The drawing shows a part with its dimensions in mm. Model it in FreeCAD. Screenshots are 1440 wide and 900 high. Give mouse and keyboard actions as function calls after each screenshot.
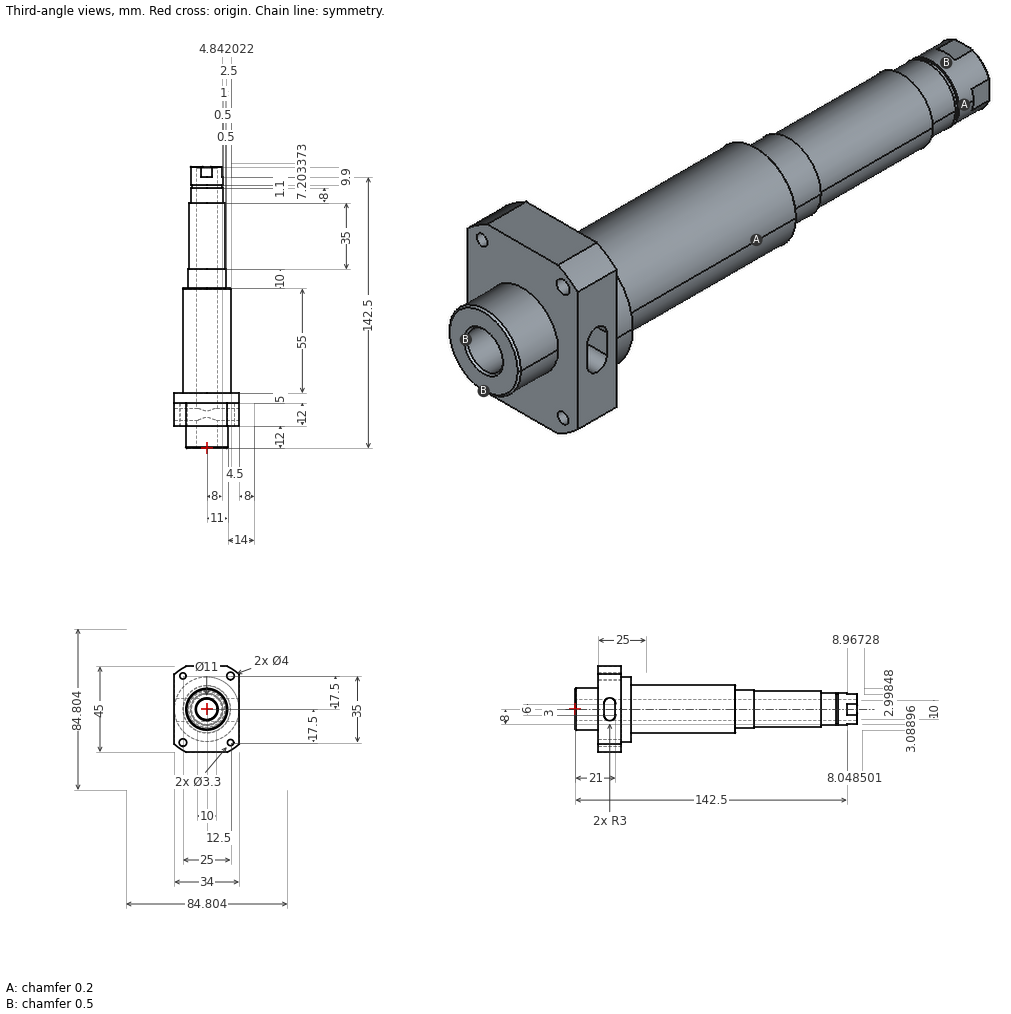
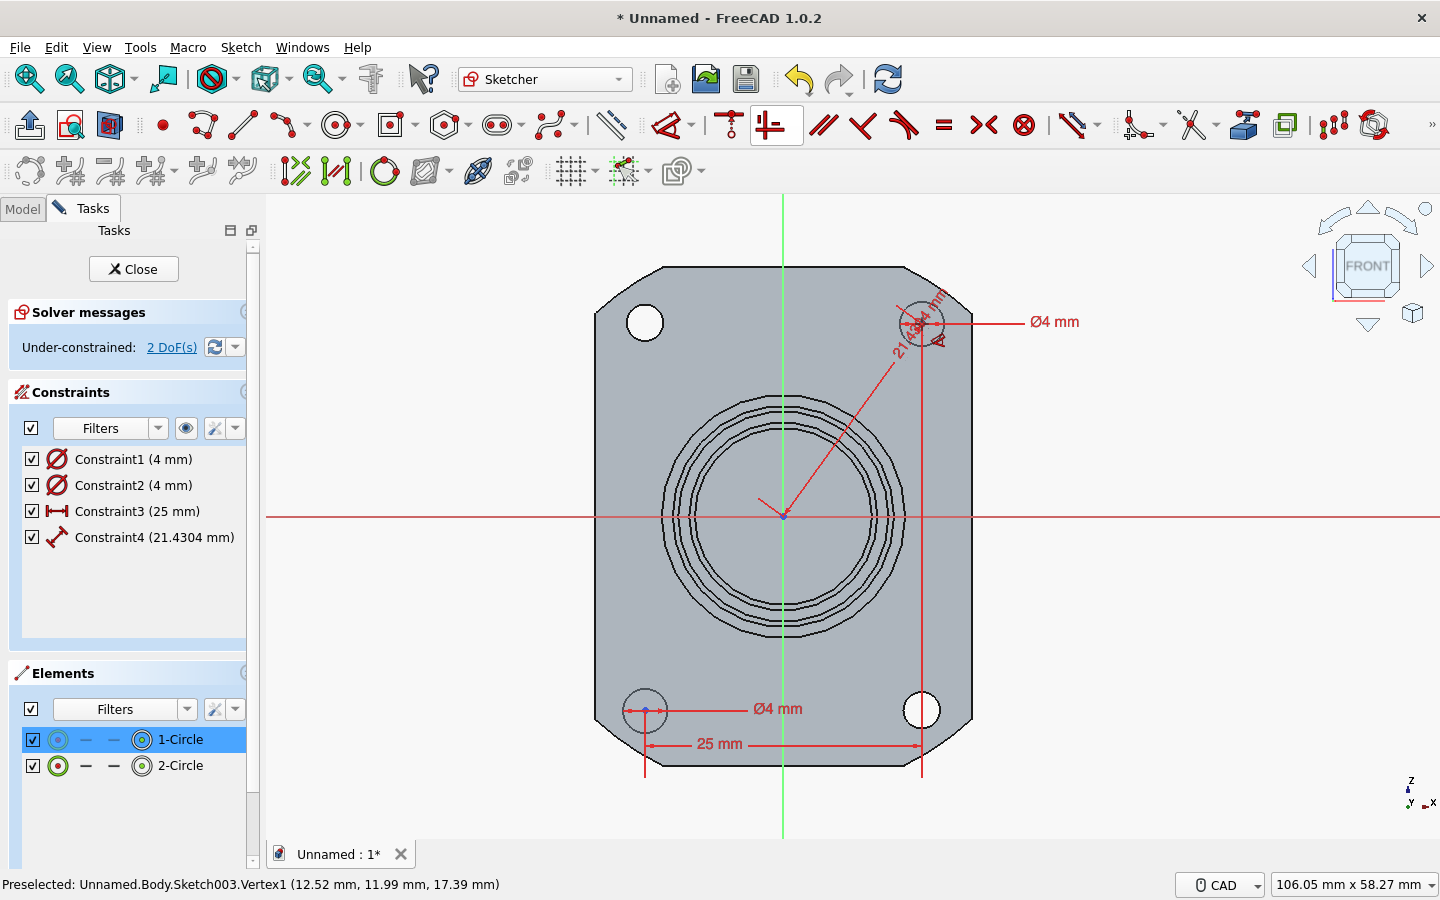
click(645, 711)
click(956, 428)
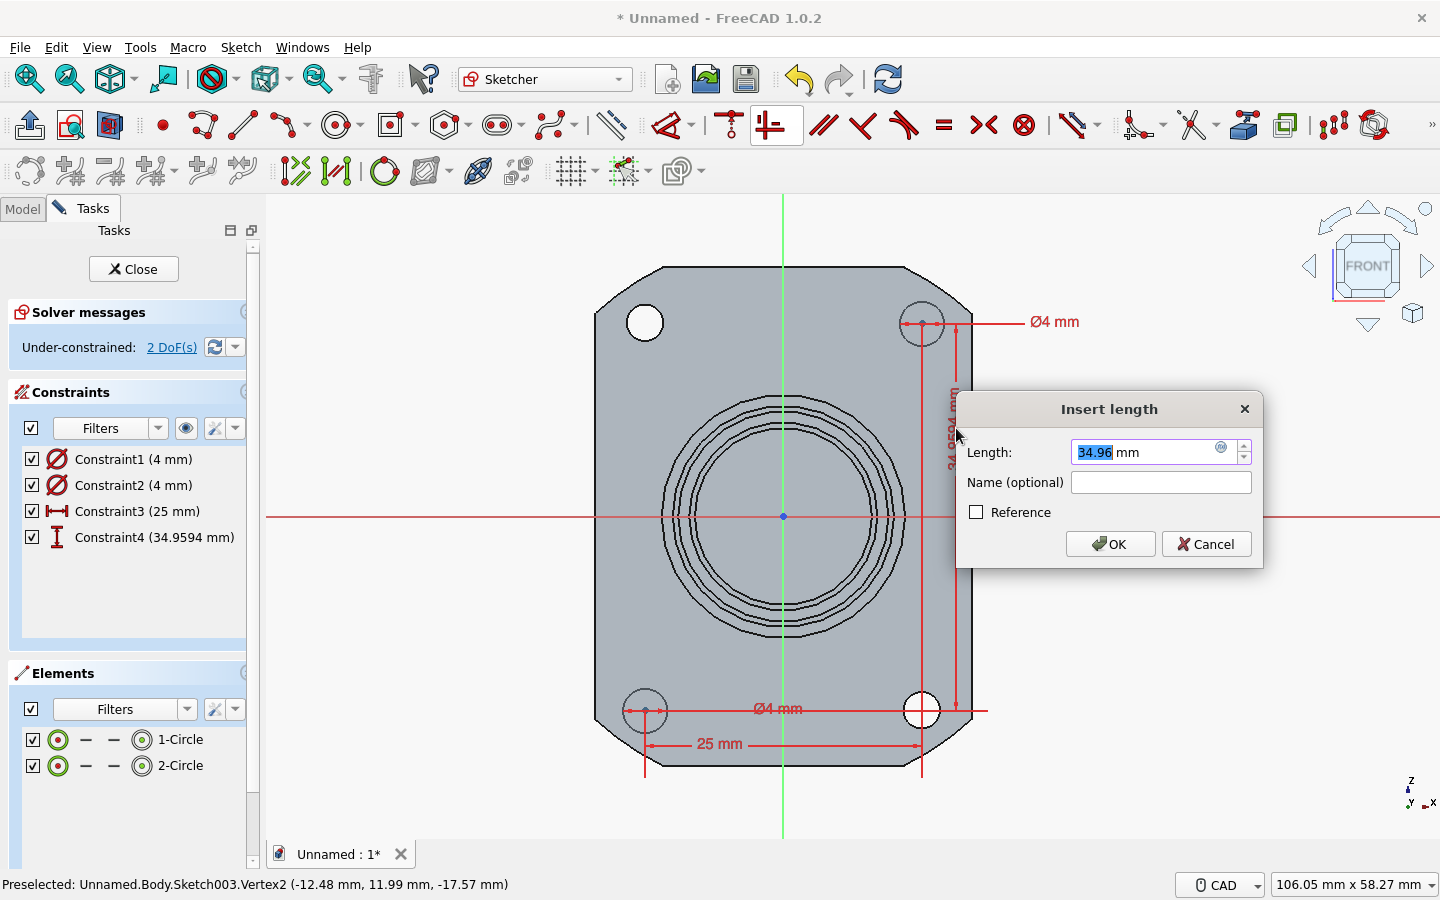
text(35)
key(Return)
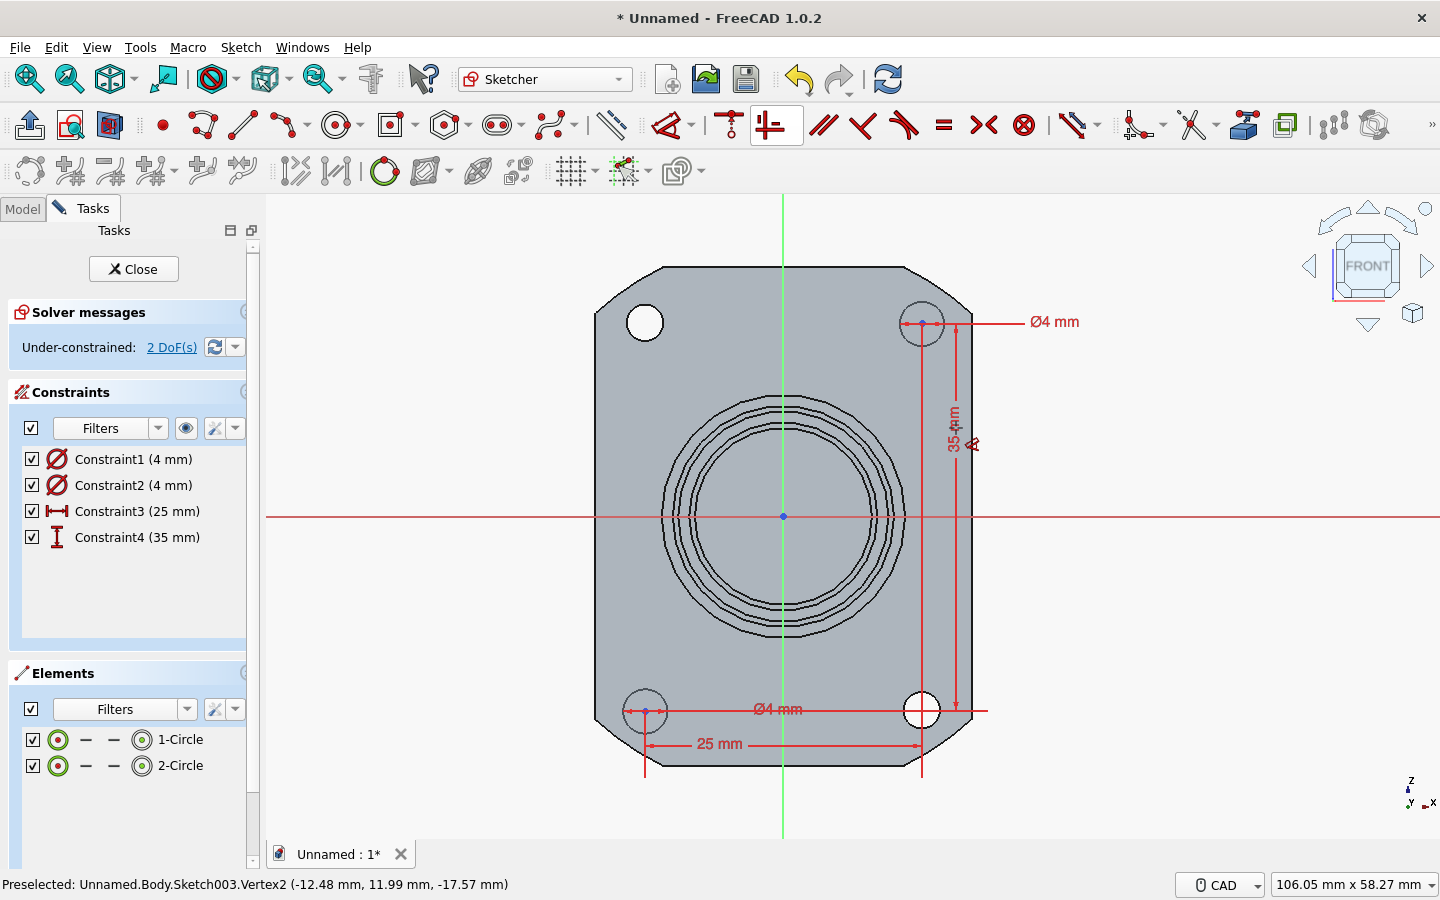
click(922, 324)
click(853, 290)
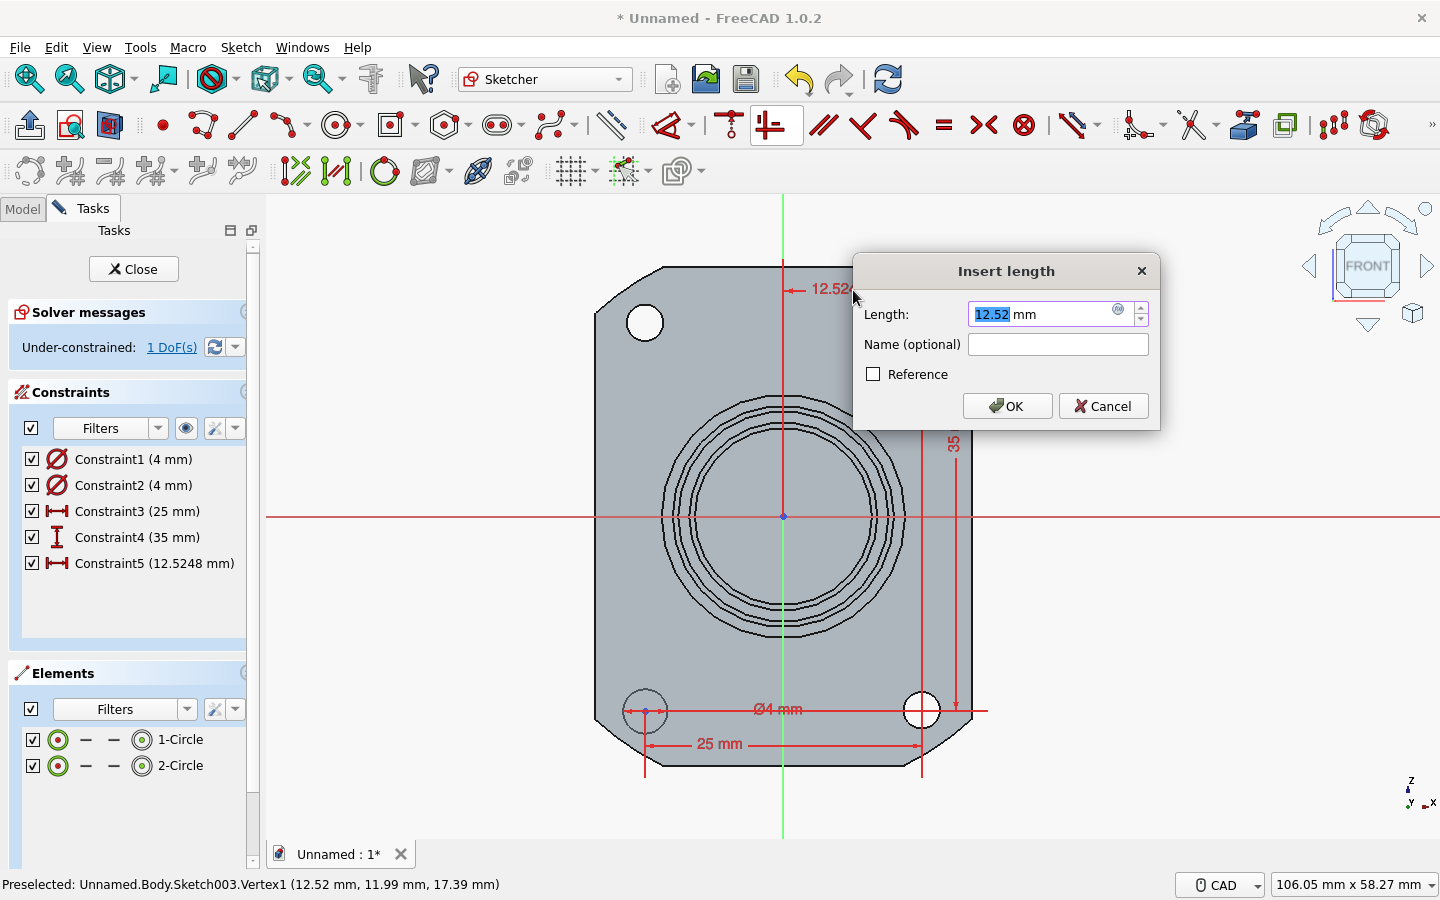
text(12.5)
key(Return)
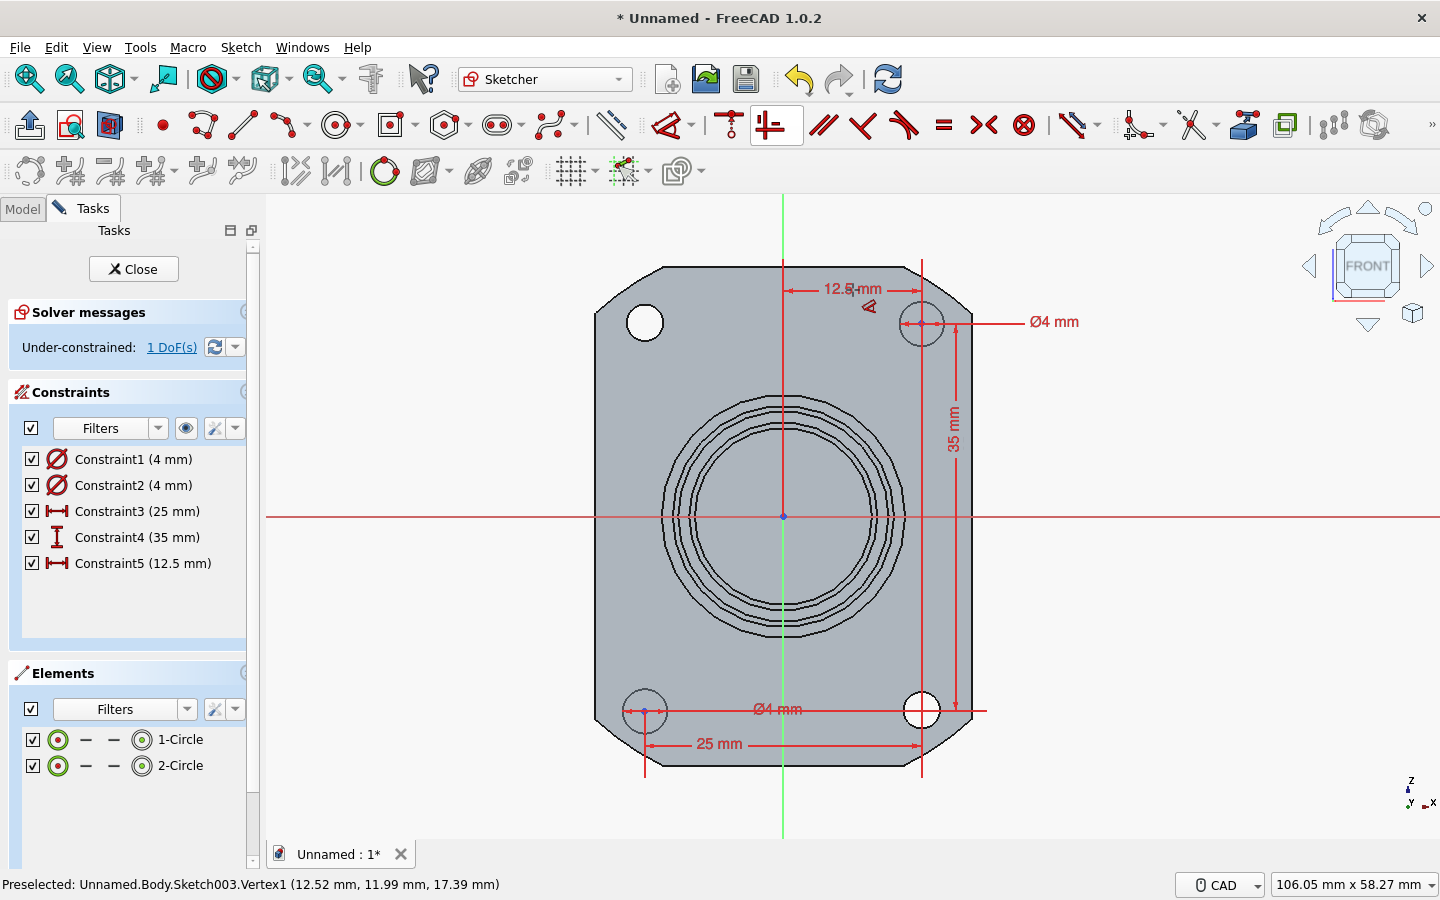
click(922, 324)
click(956, 376)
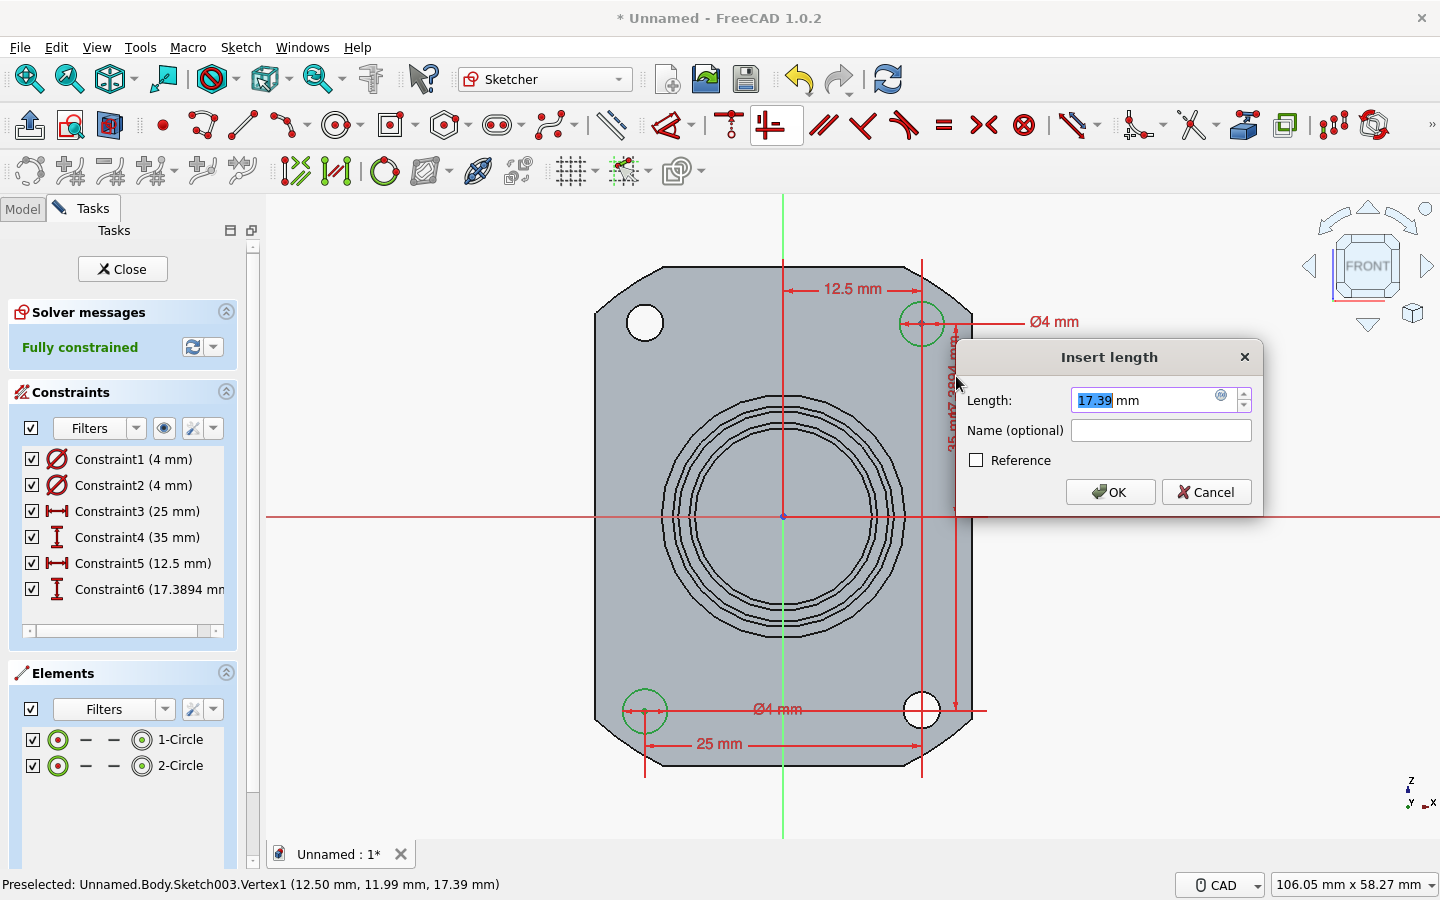
text(17.5)
key(Return)
key(Escape)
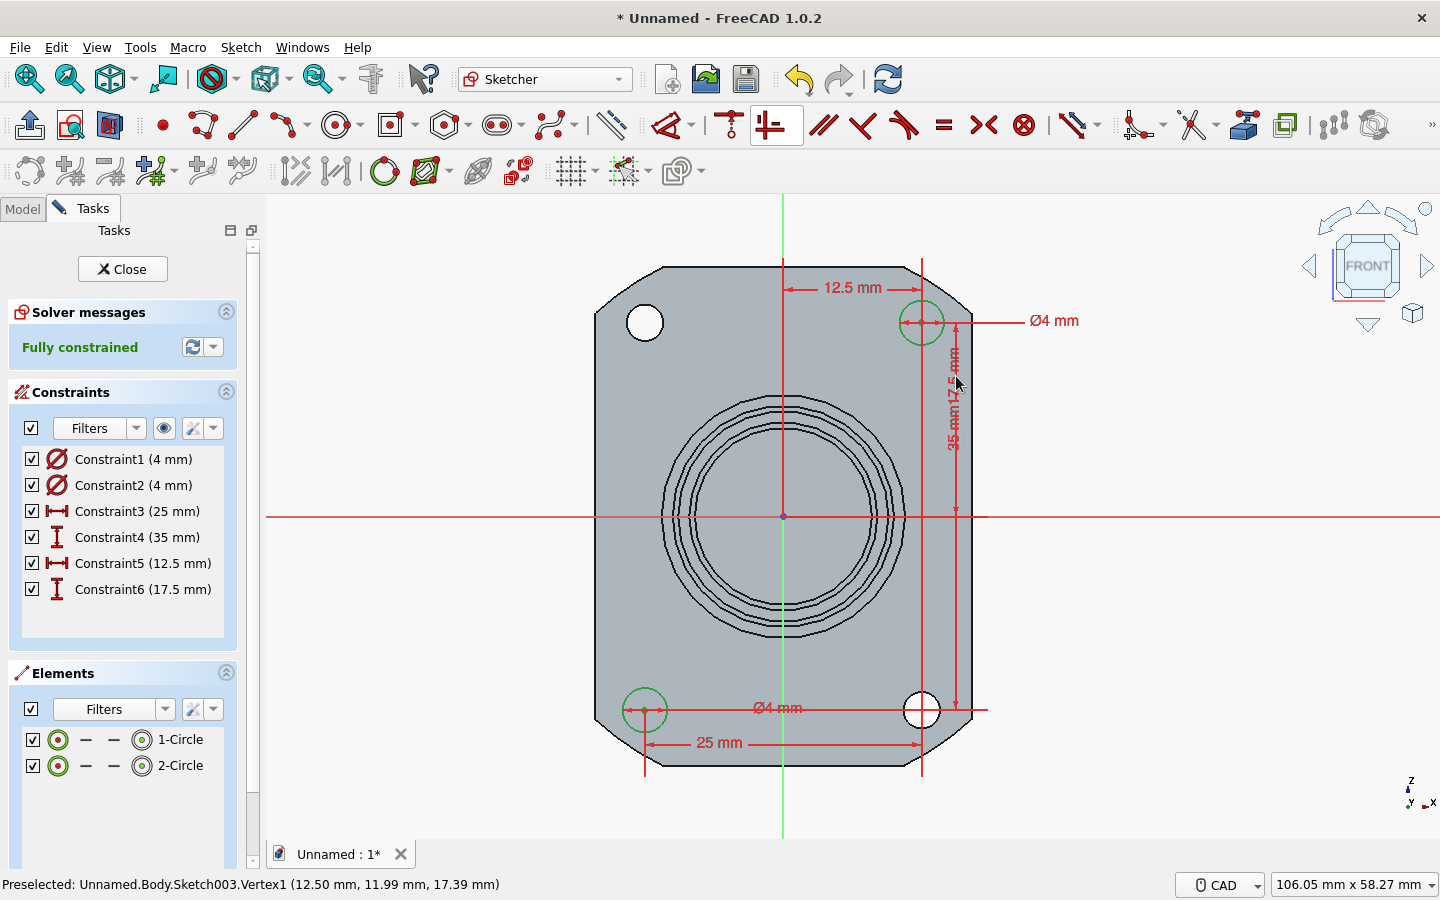
click(123, 269)